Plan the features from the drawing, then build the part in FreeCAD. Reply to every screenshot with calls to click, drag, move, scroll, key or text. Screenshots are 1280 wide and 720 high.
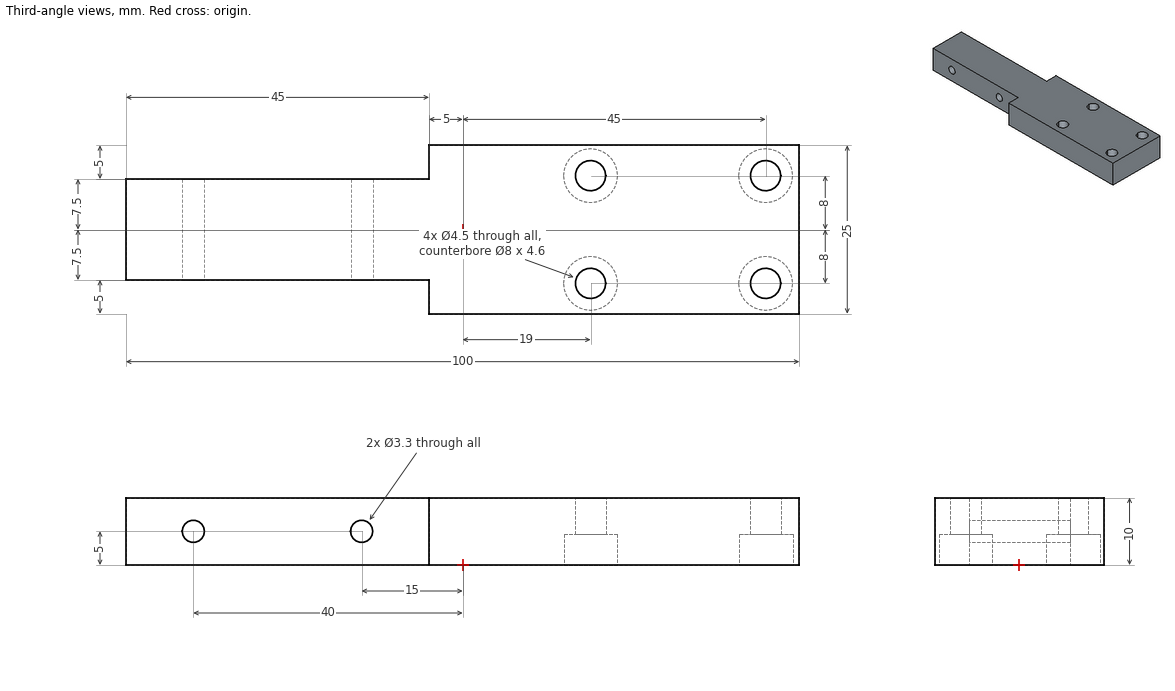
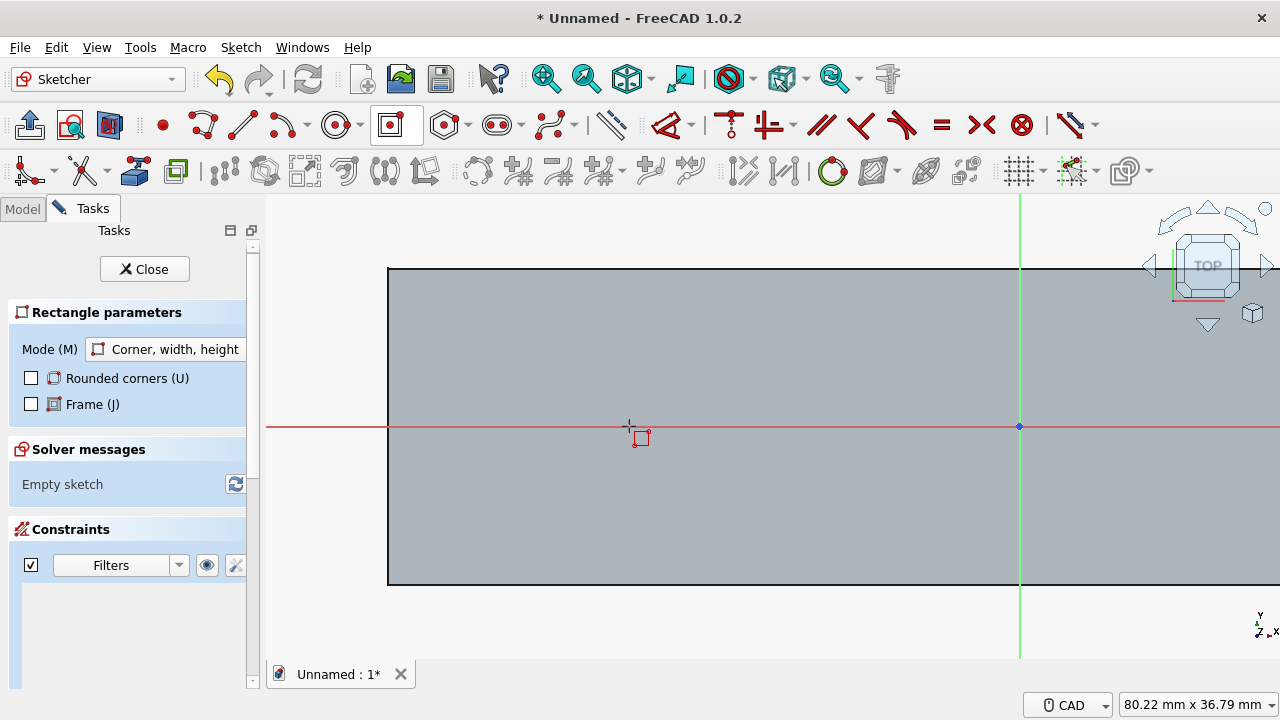
click(388, 268)
click(957, 332)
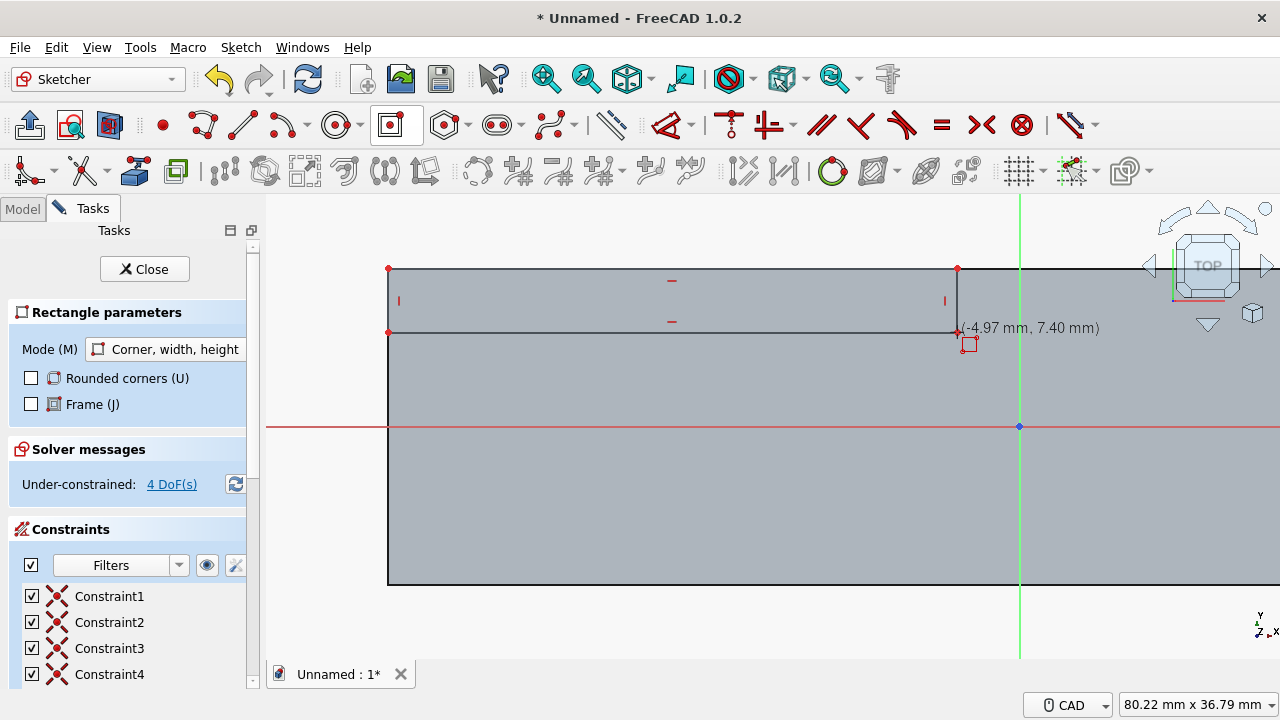
click(388, 521)
click(957, 585)
key(Escape)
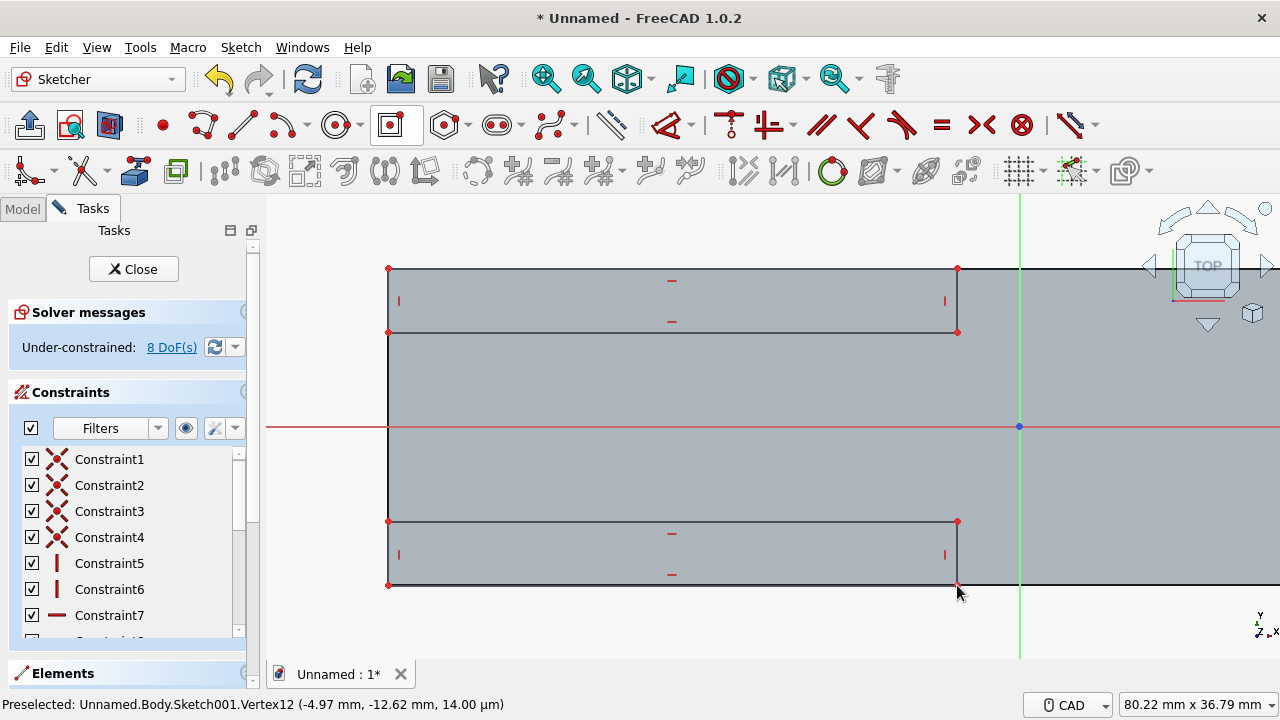
click(666, 126)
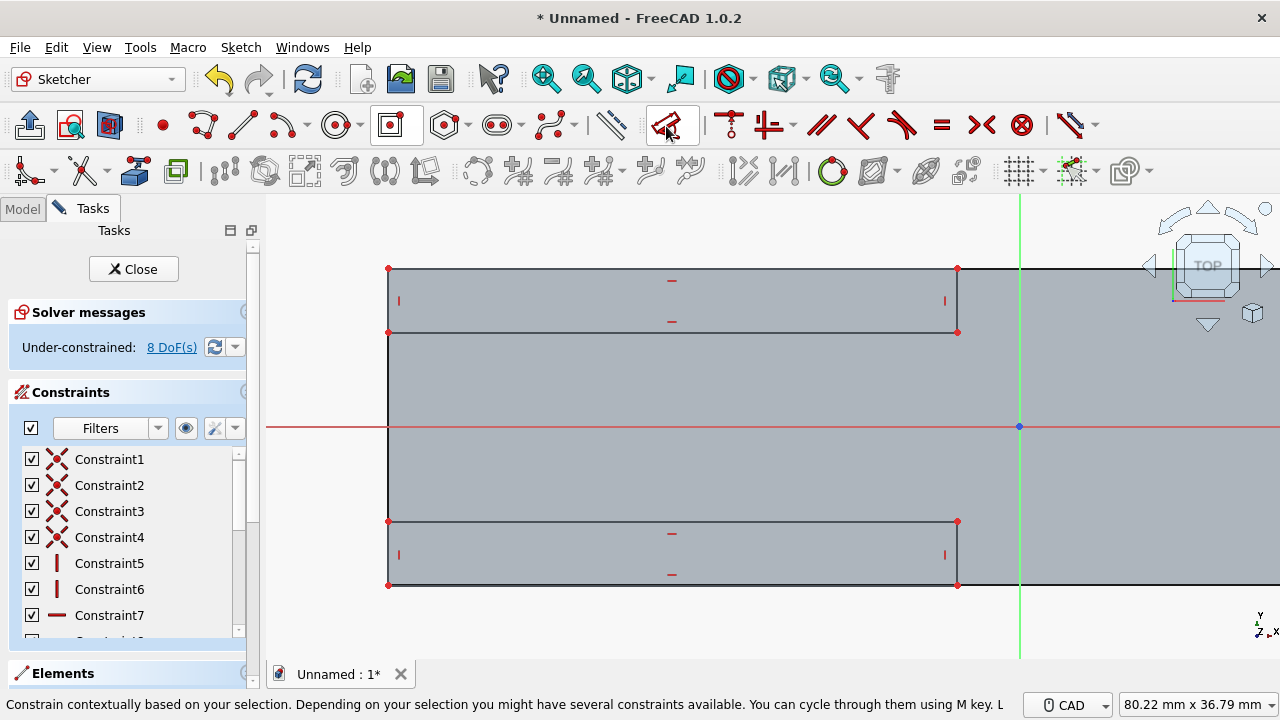
click(388, 288)
click(354, 301)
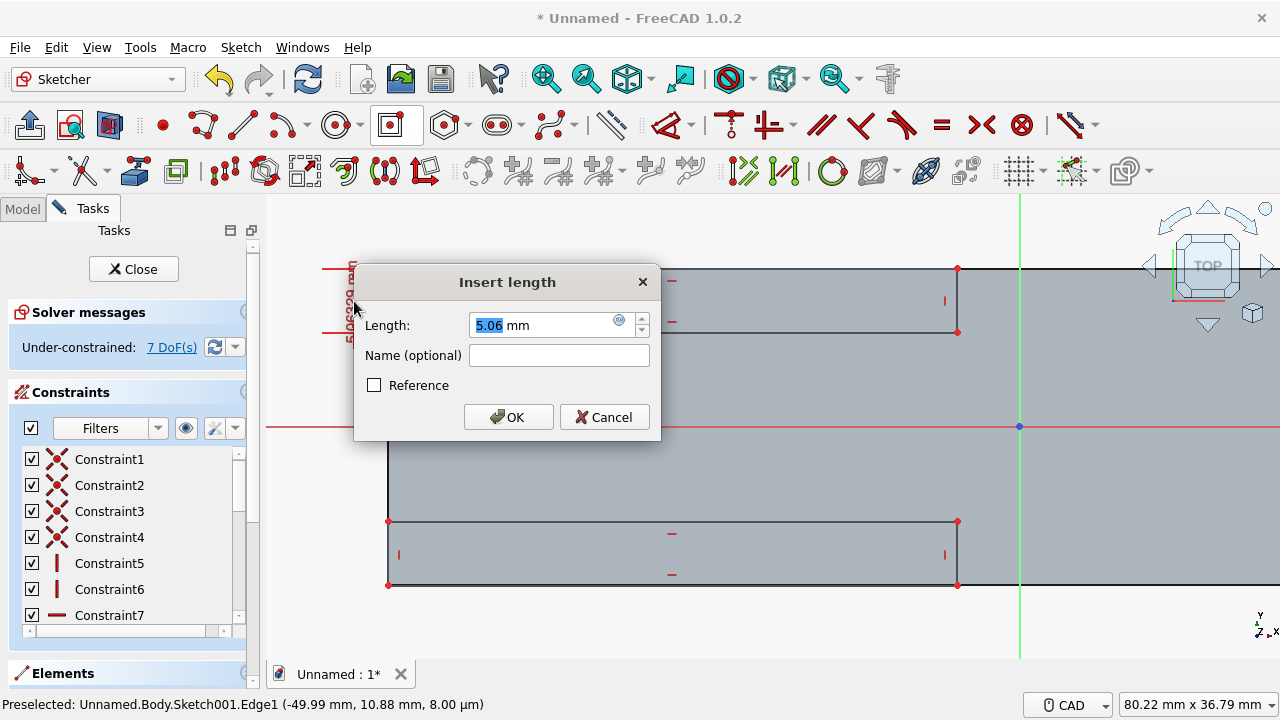
text(5)
key(Return)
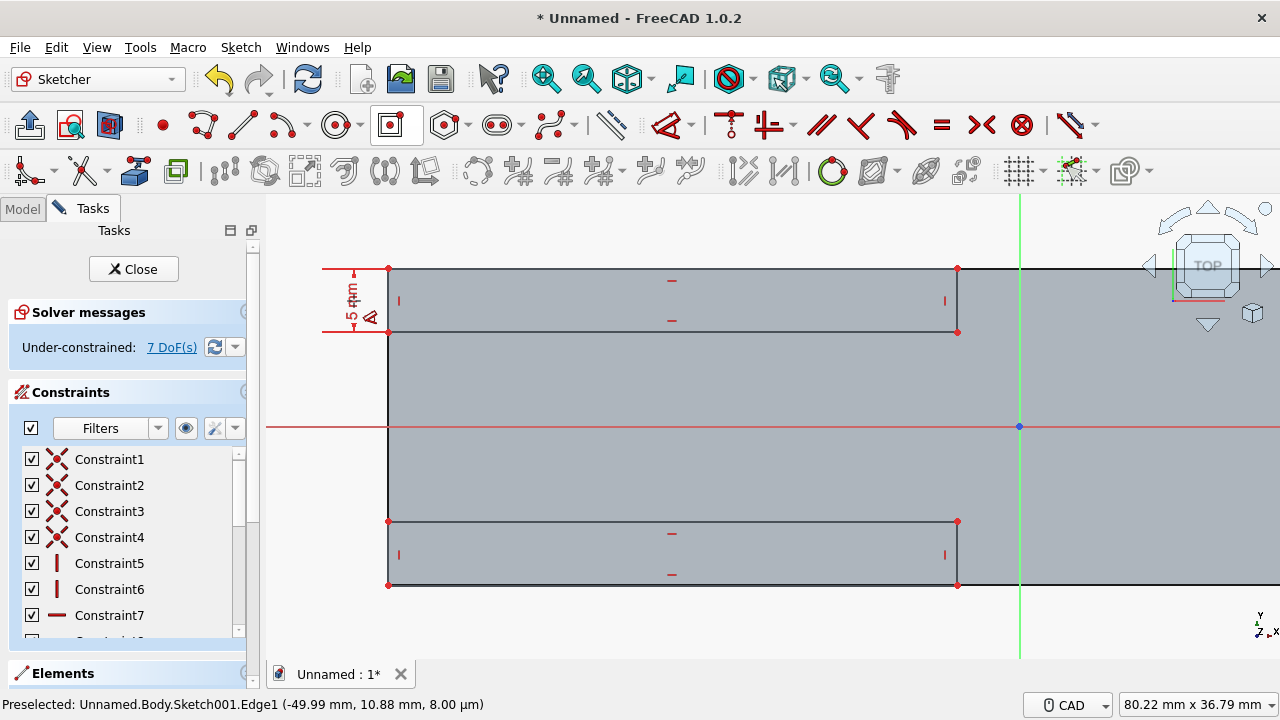
click(388, 541)
click(354, 554)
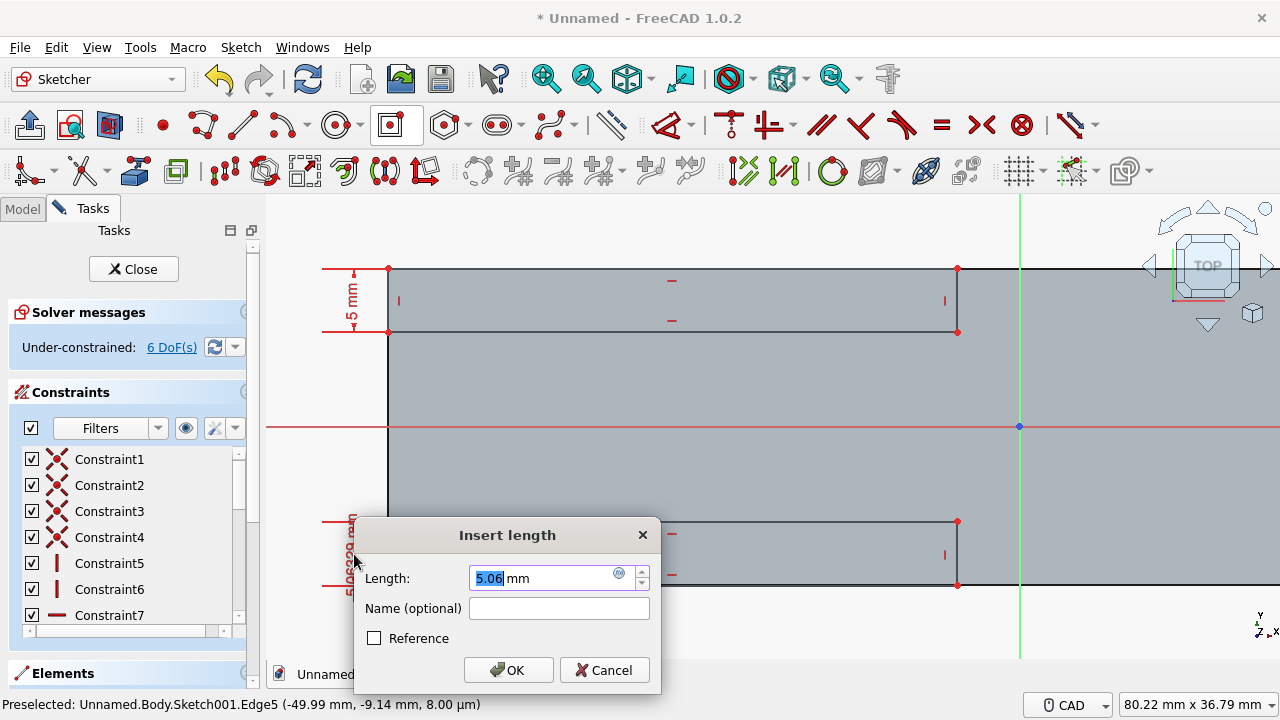
text(5)
key(Return)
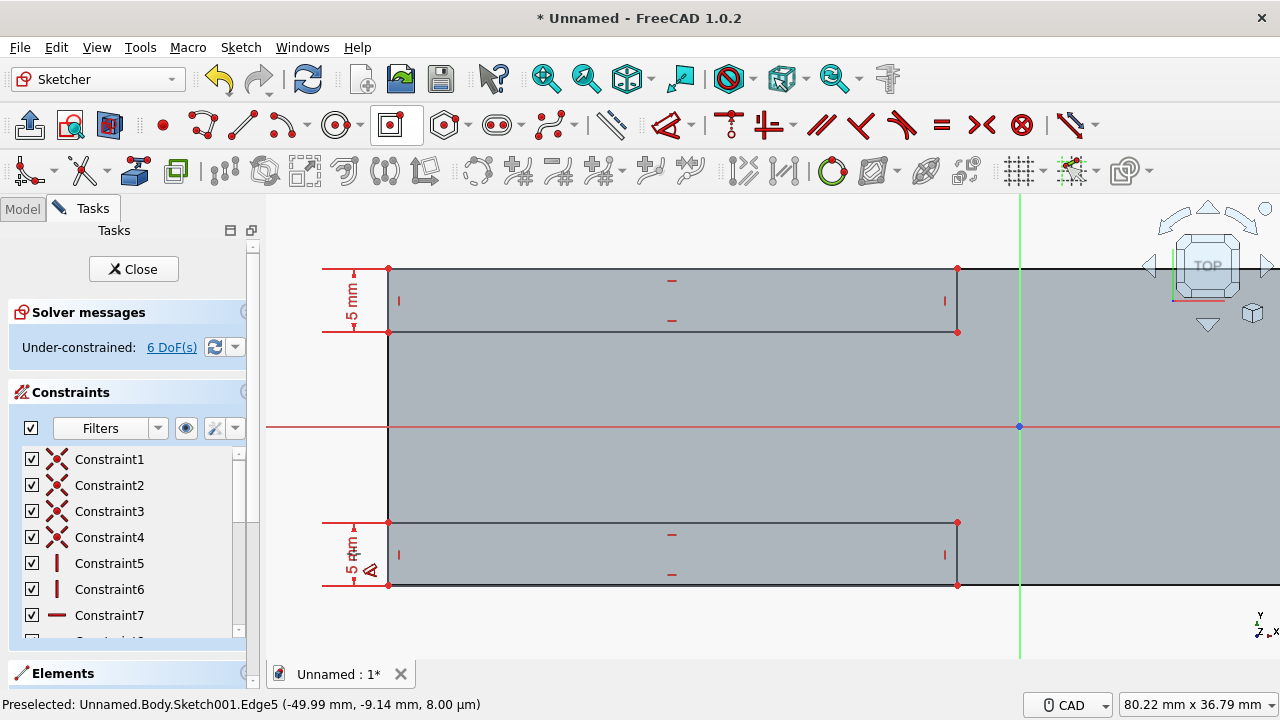
click(559, 332)
click(672, 298)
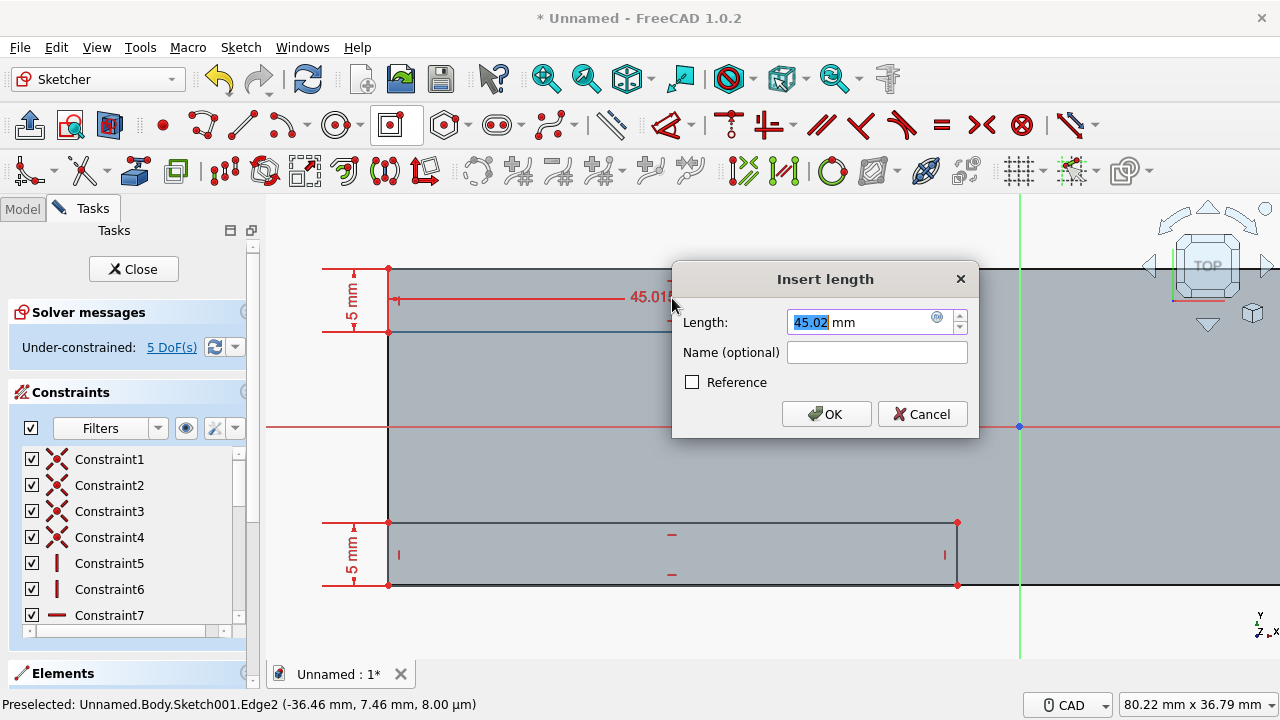
text(45)
key(Return)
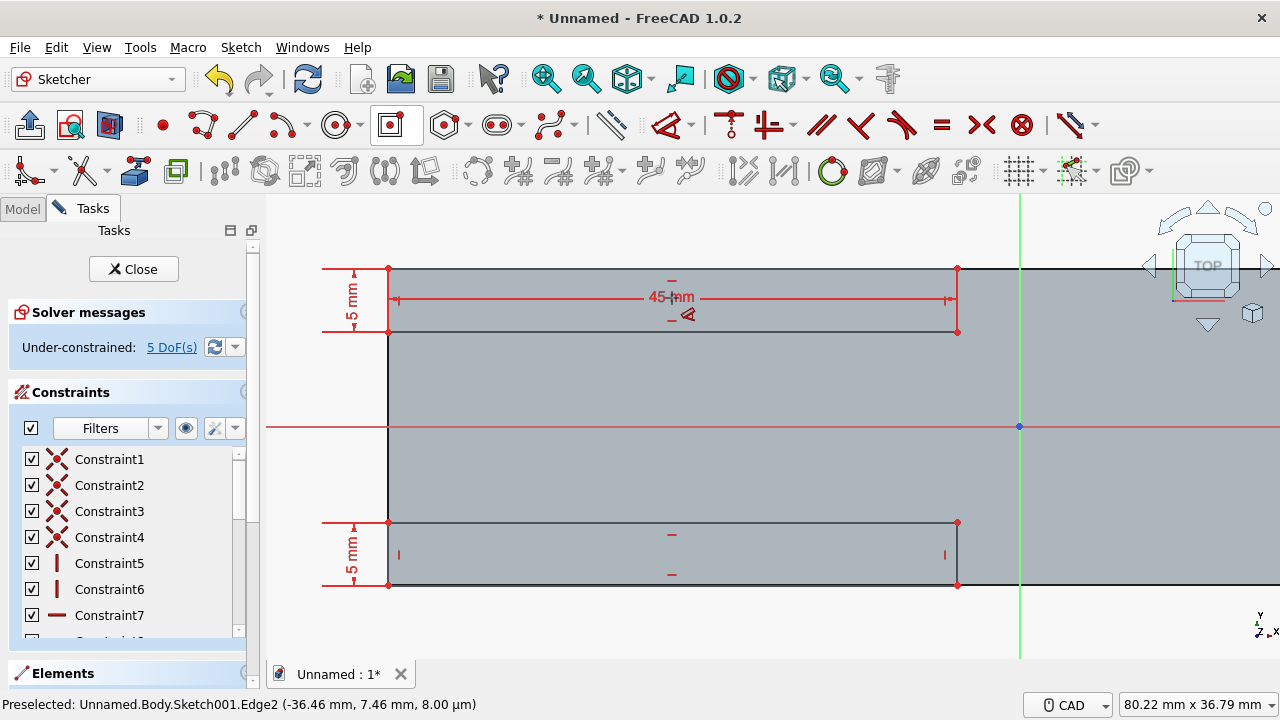
click(559, 586)
click(672, 620)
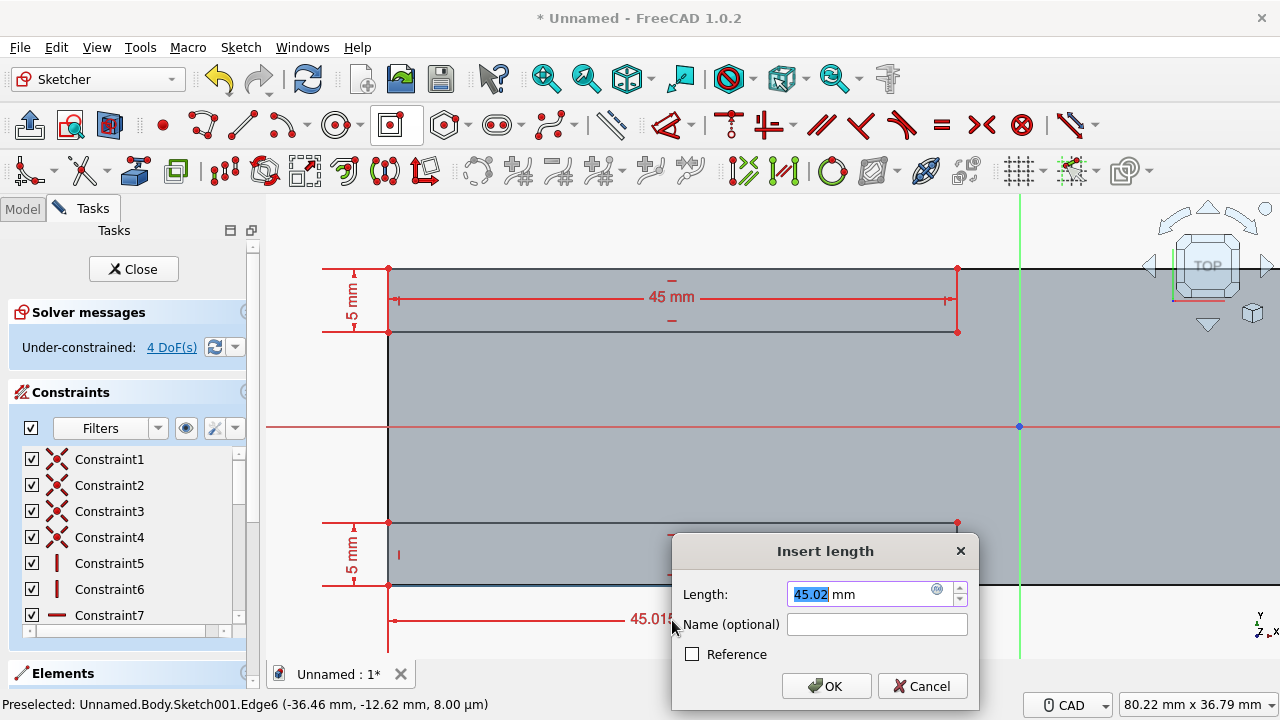
text(45)
key(Return)